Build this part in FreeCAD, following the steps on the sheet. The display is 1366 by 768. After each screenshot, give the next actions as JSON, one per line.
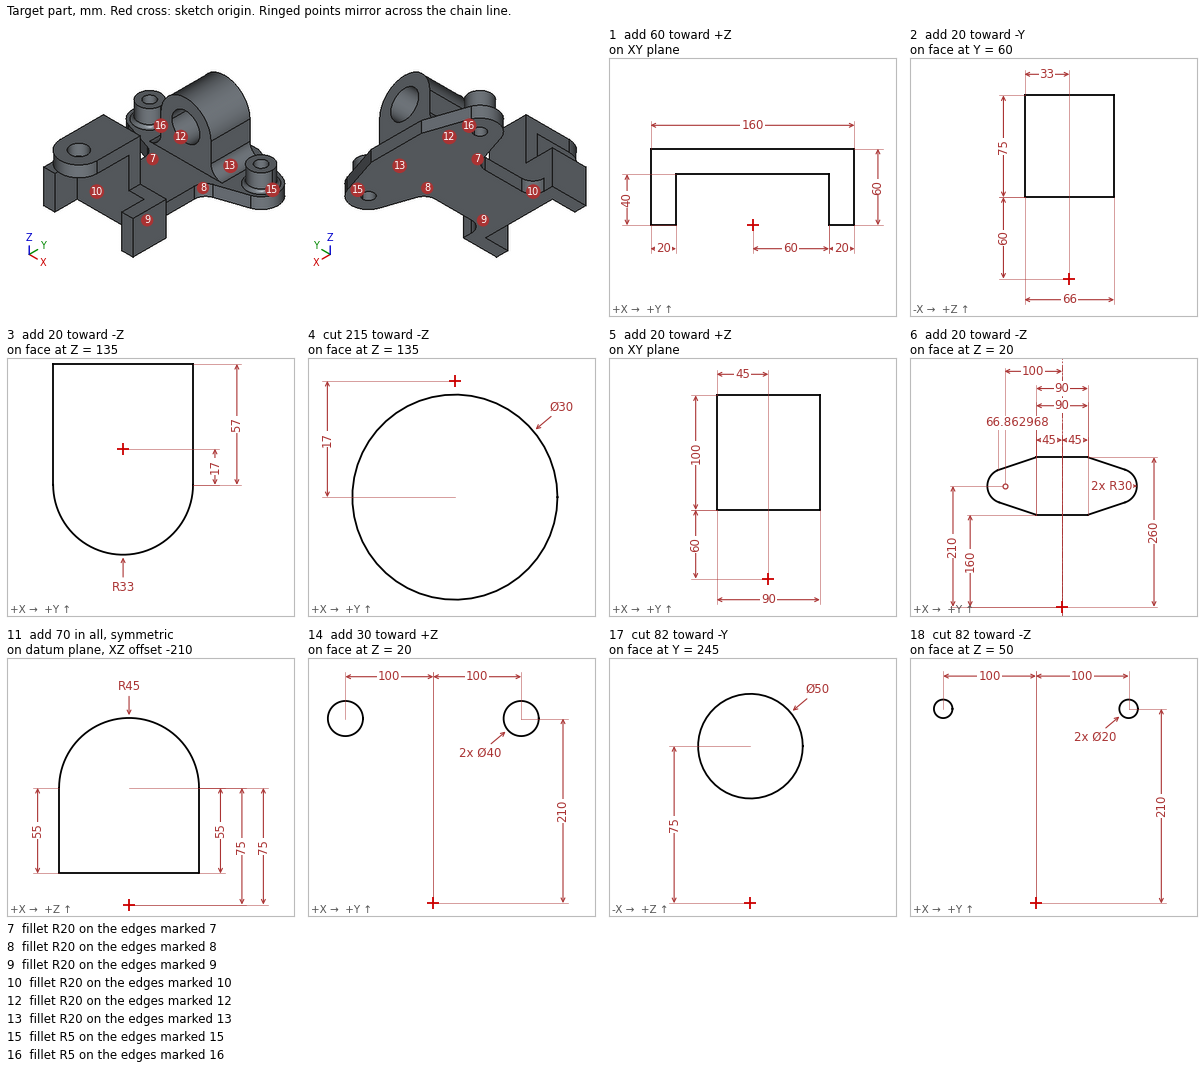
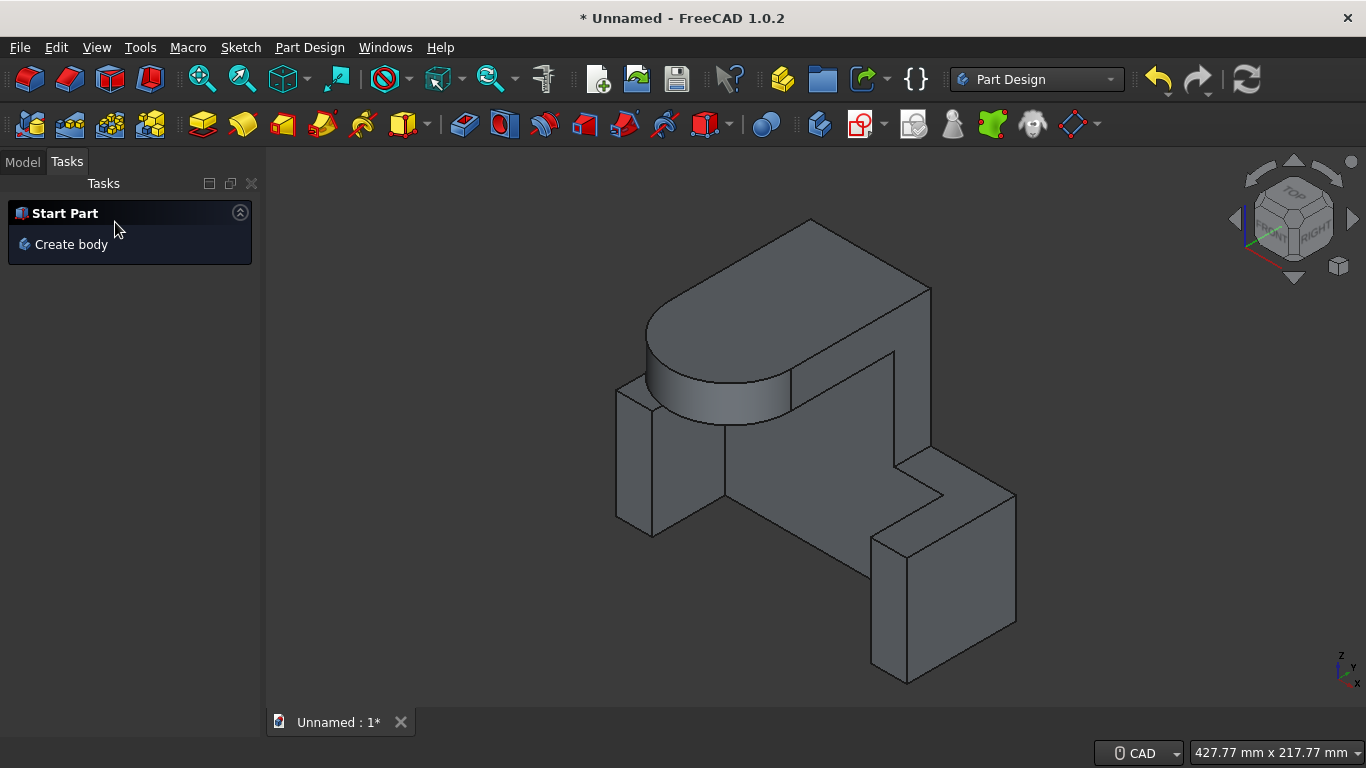
{"action": "key", "text": "v f"}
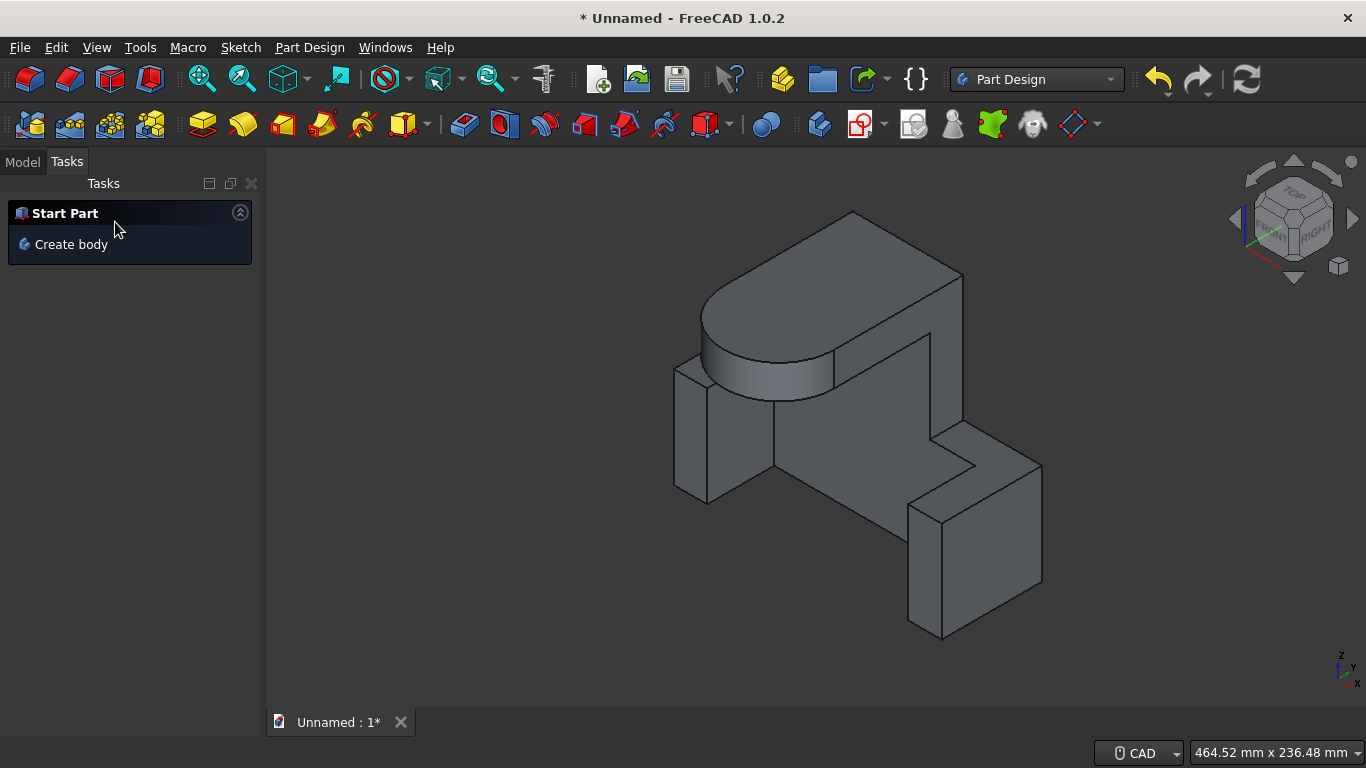
{"action": "left_click", "coordinate": [842, 280]}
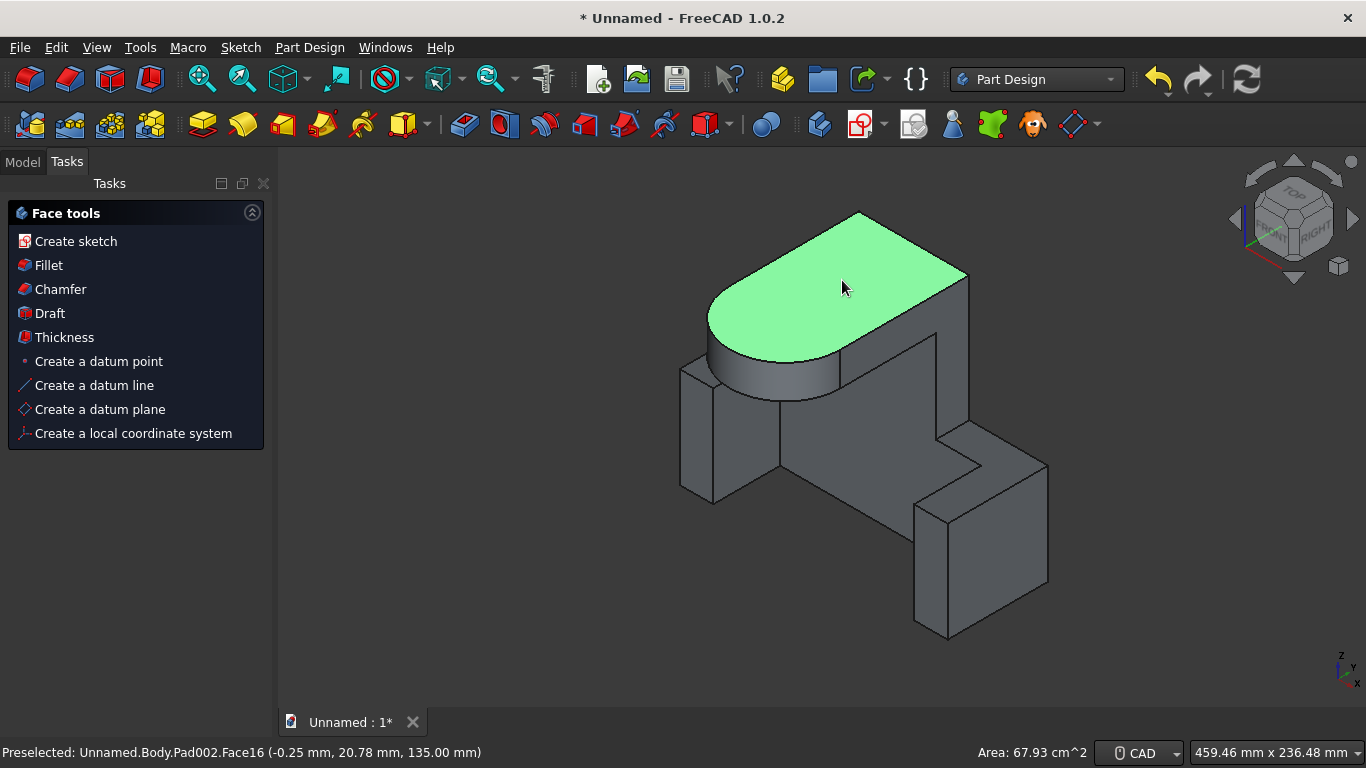
{"action": "left_click", "coordinate": [860, 124]}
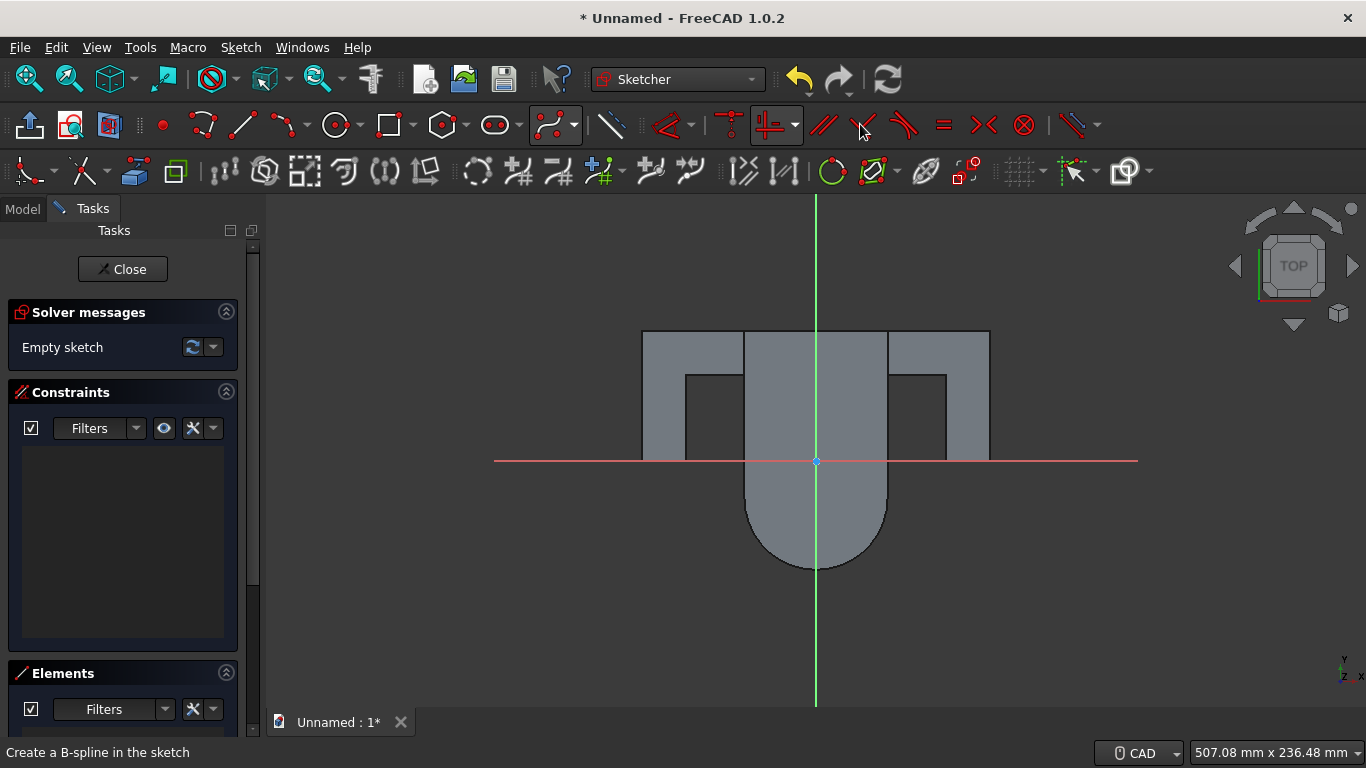
{"action": "scroll", "coordinate": [833, 508], "scroll_direction": "up", "scroll_amount": 8}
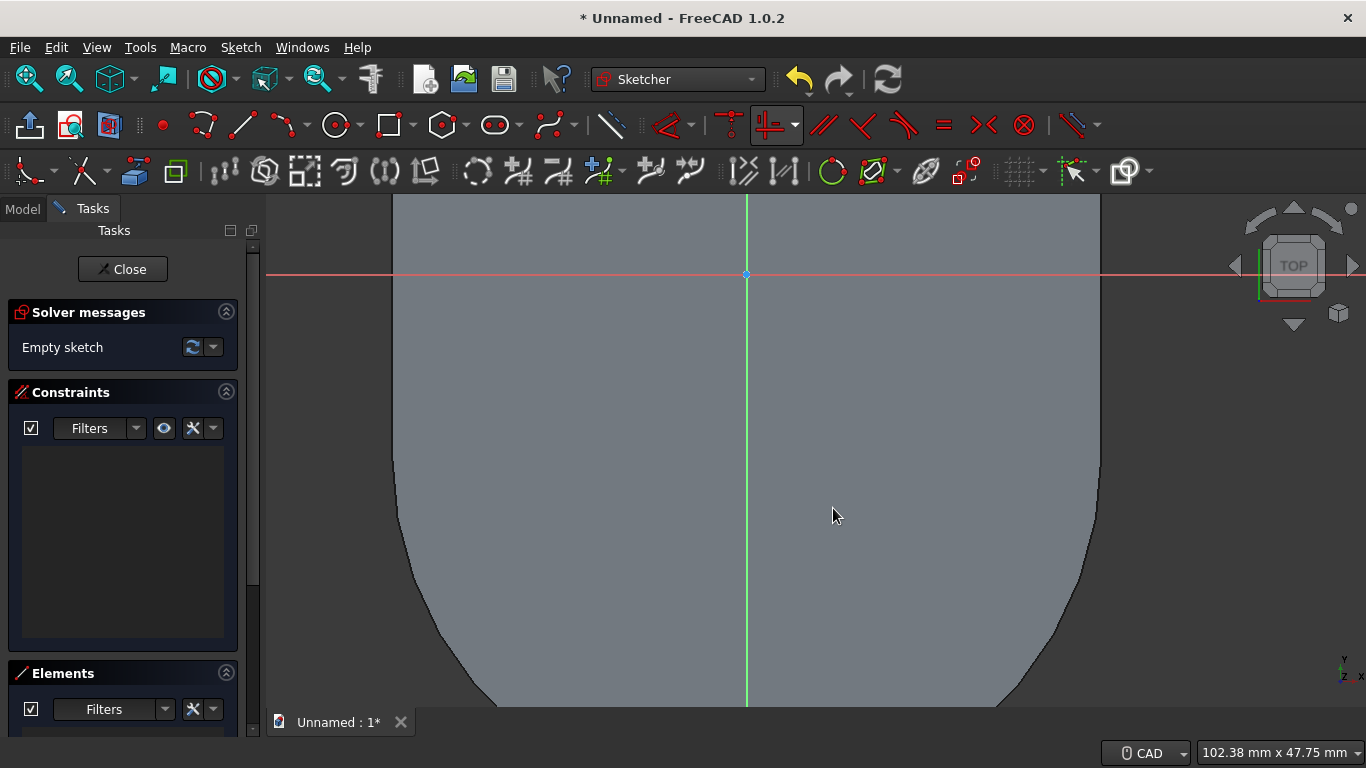
{"action": "key", "text": "g c"}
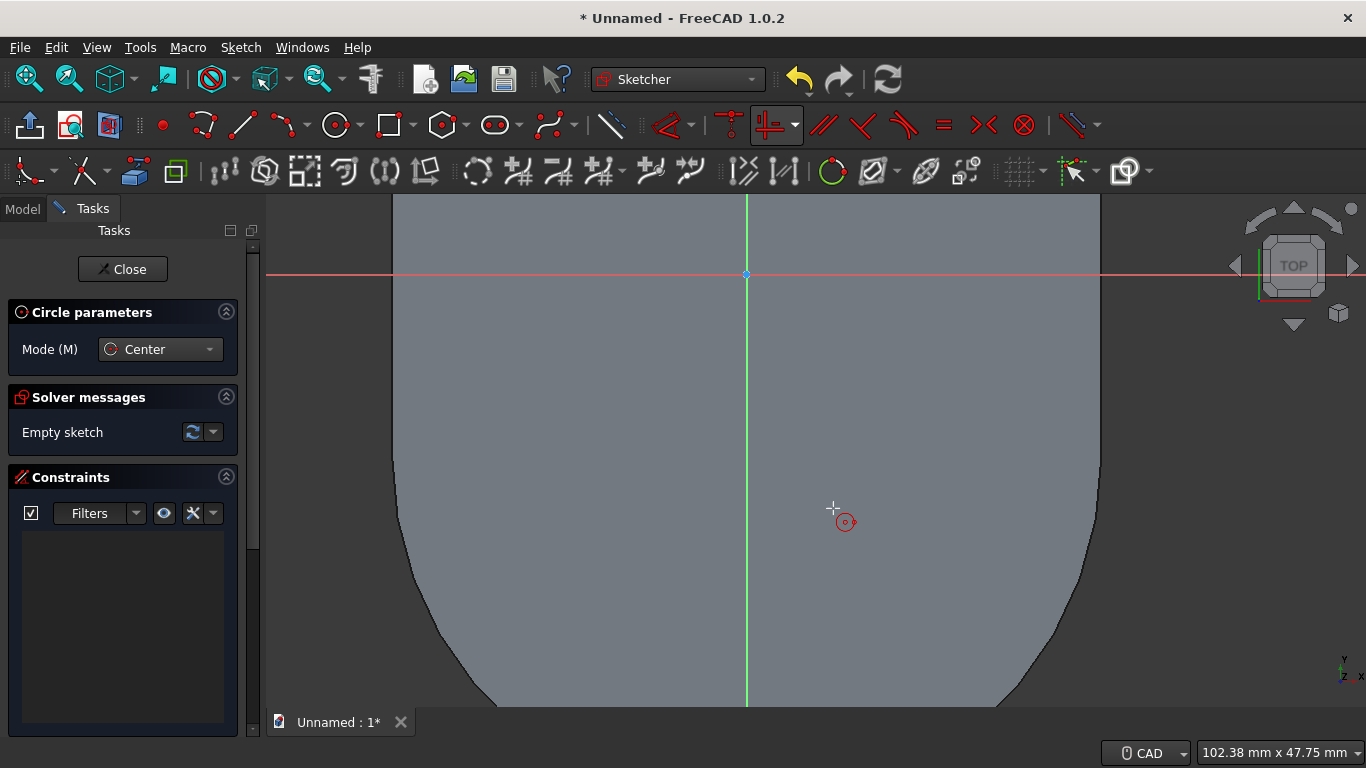
{"action": "left_click", "coordinate": [747, 457]}
{"action": "left_click", "coordinate": [861, 343]}
{"action": "key", "text": "Escape"}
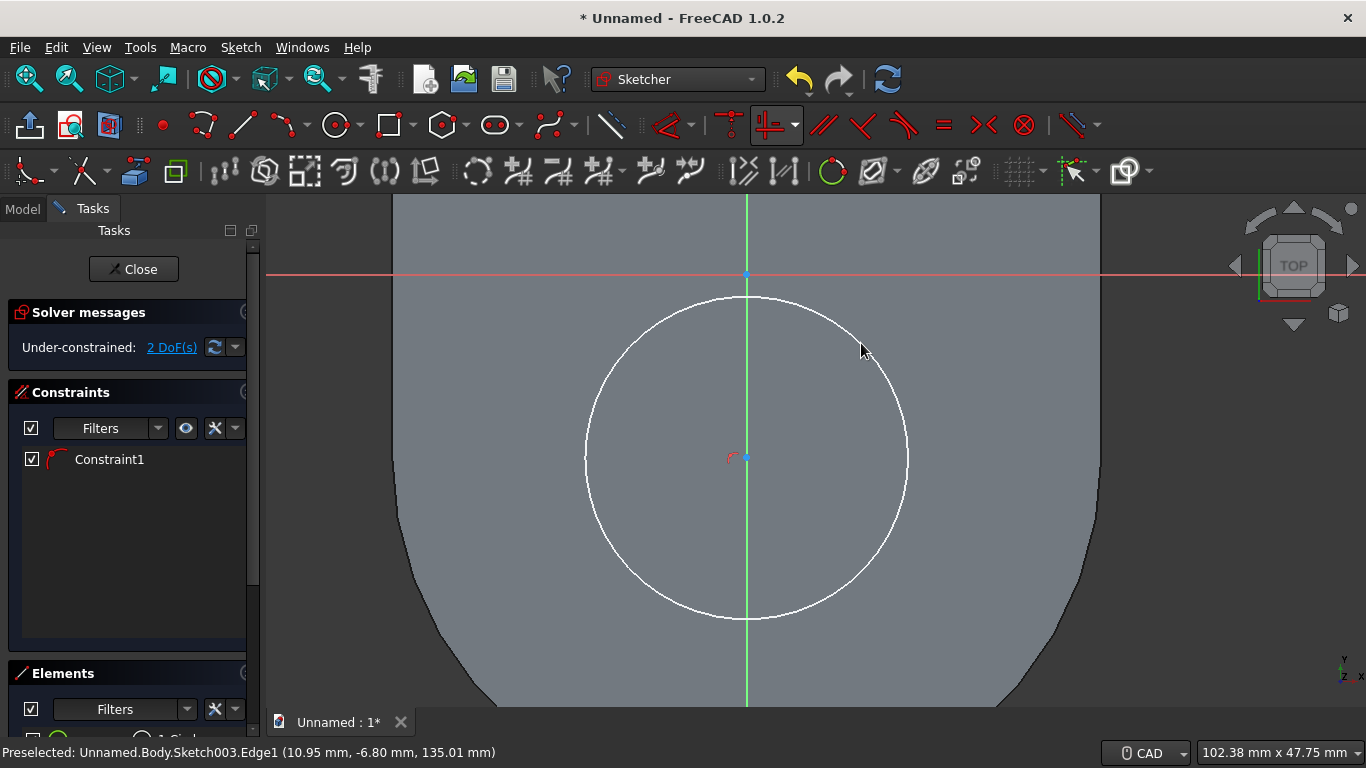
{"action": "key", "text": "d"}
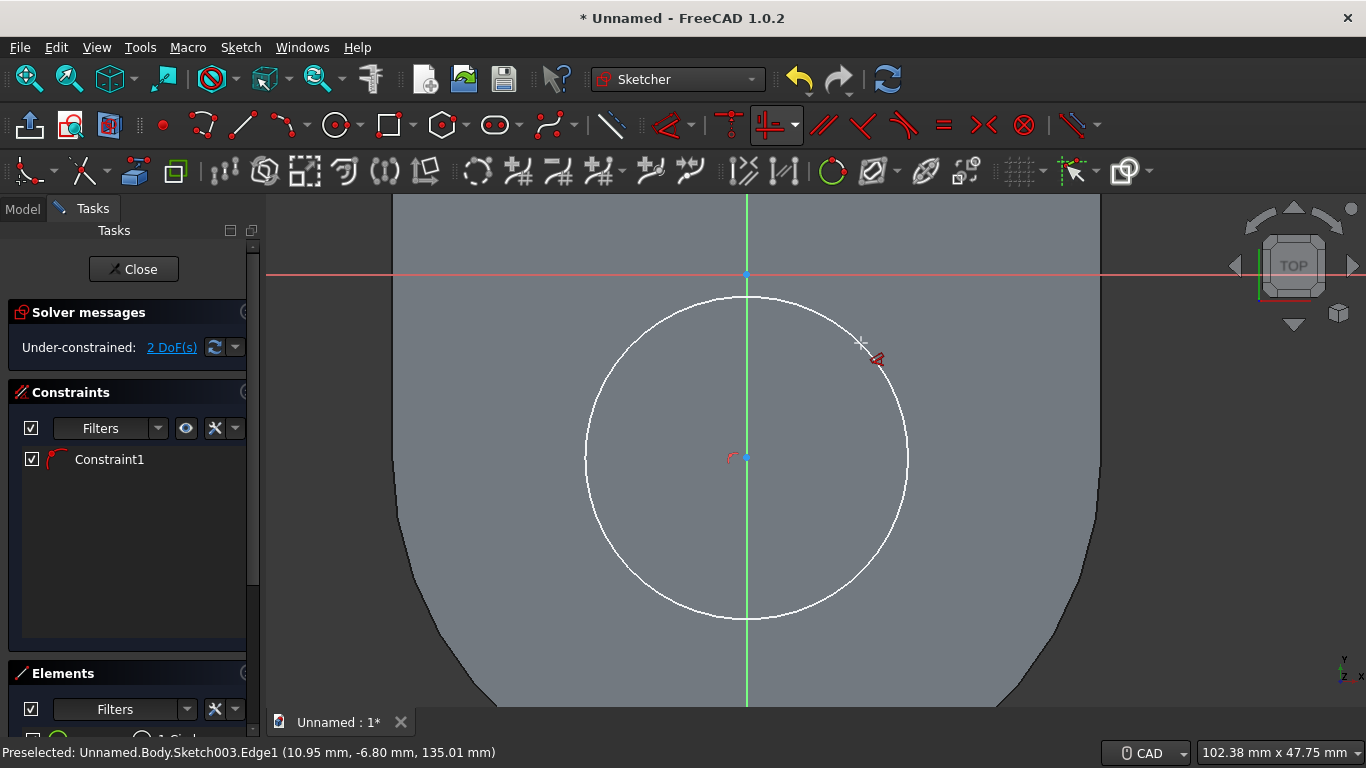
{"action": "left_click", "coordinate": [861, 344]}
{"action": "left_click", "coordinate": [884, 321]}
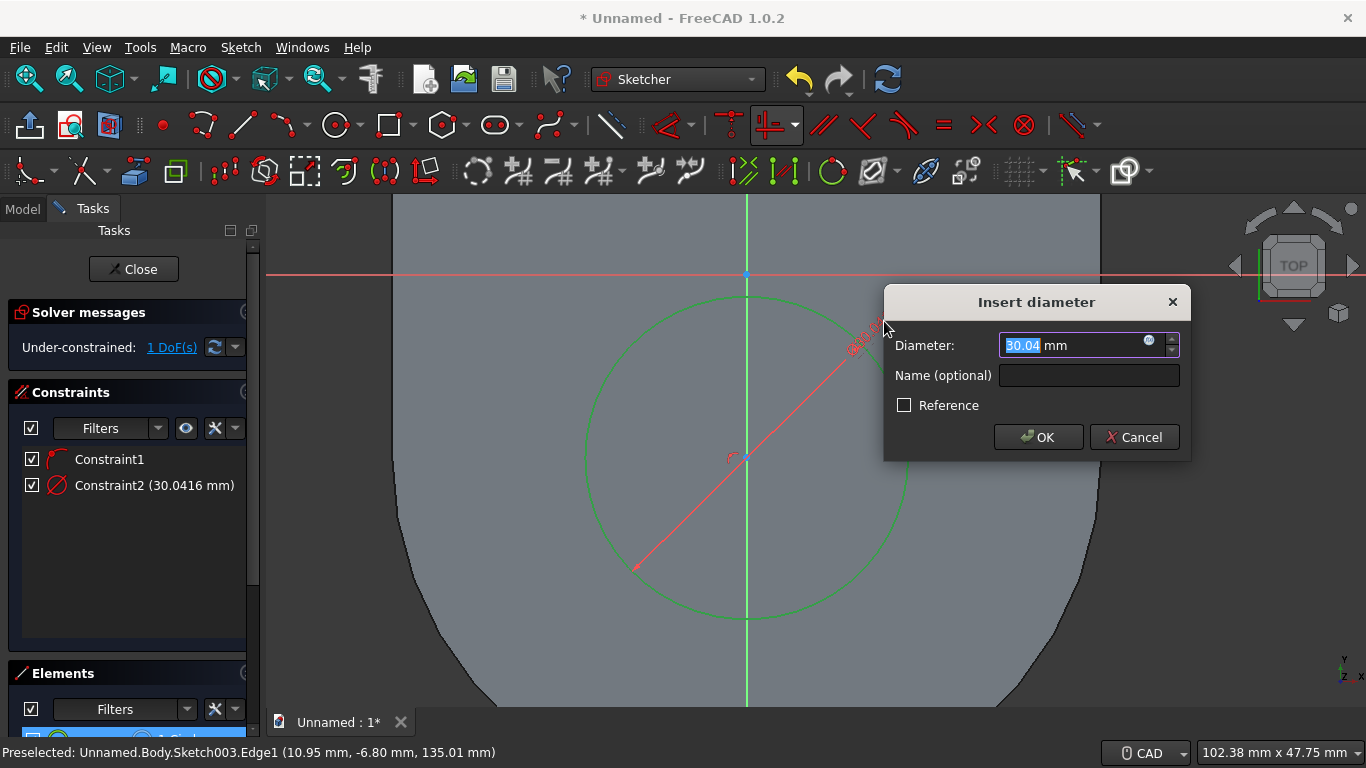
{"action": "type", "text": "30"}
{"action": "key", "text": "Return"}